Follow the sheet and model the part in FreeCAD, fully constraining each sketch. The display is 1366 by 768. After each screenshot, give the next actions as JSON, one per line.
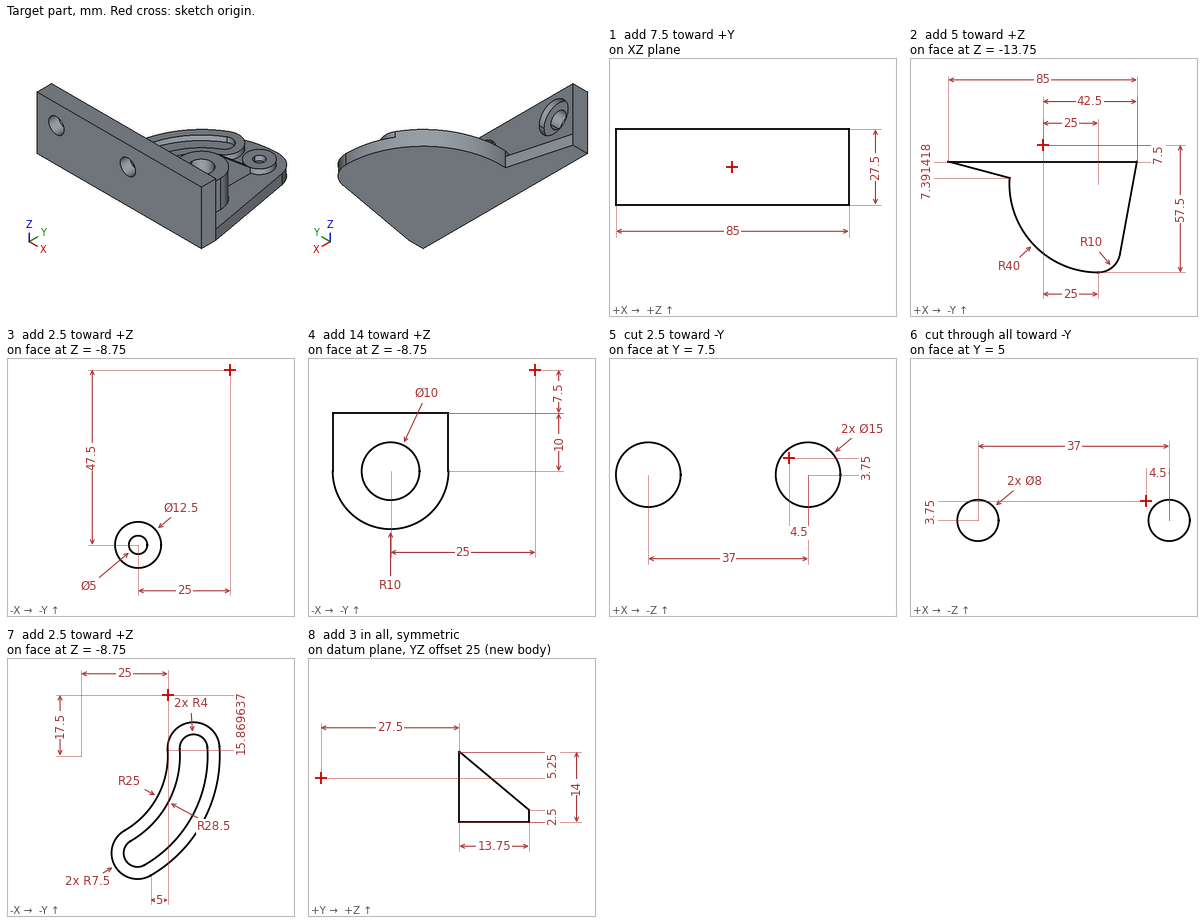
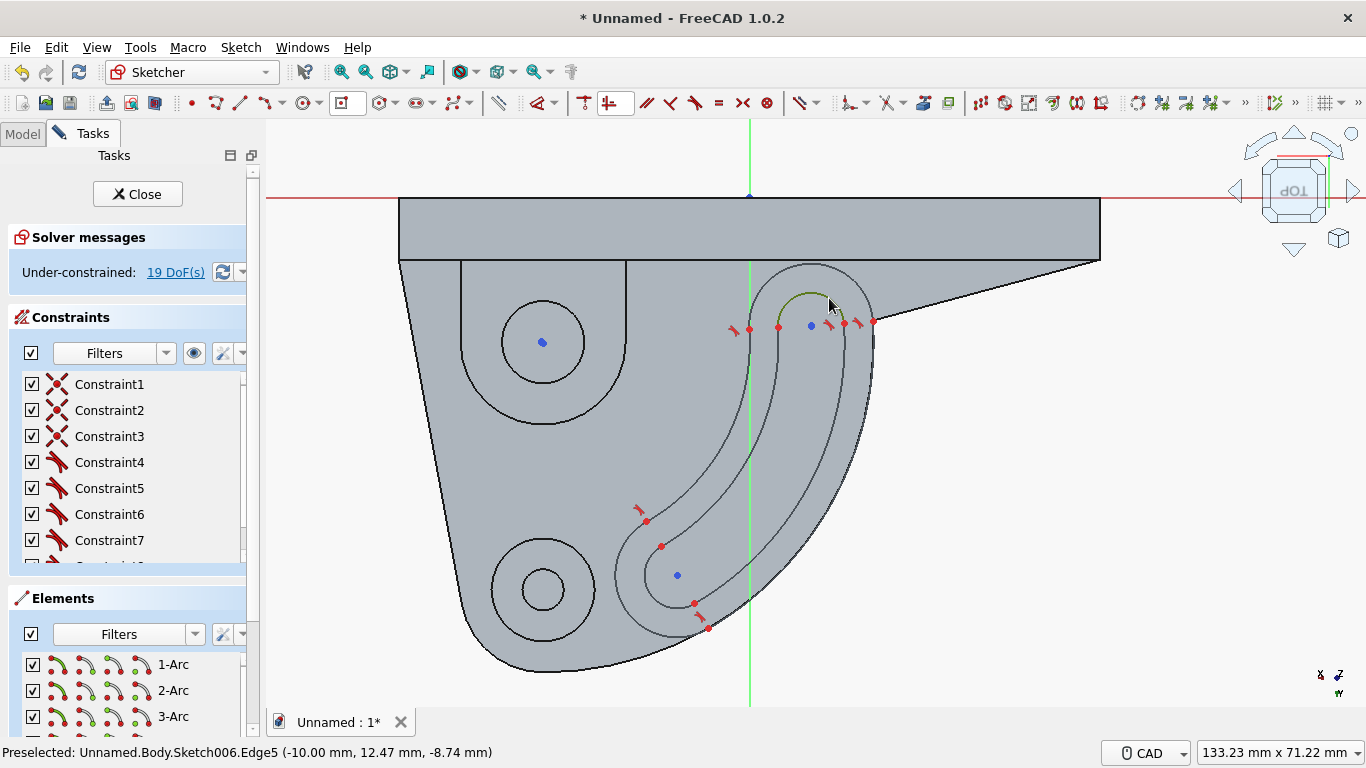
{"action": "left_click", "coordinate": [721, 497]}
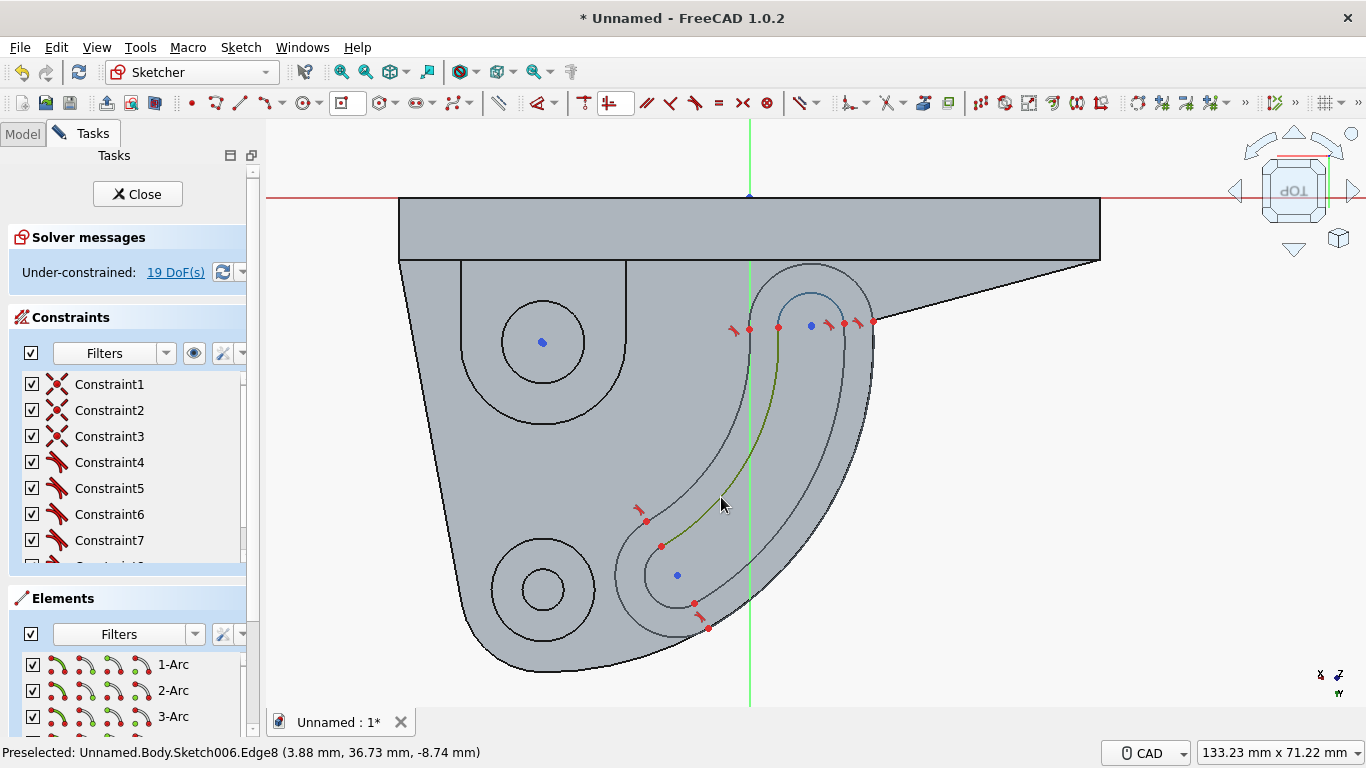
{"action": "left_click", "coordinate": [696, 104]}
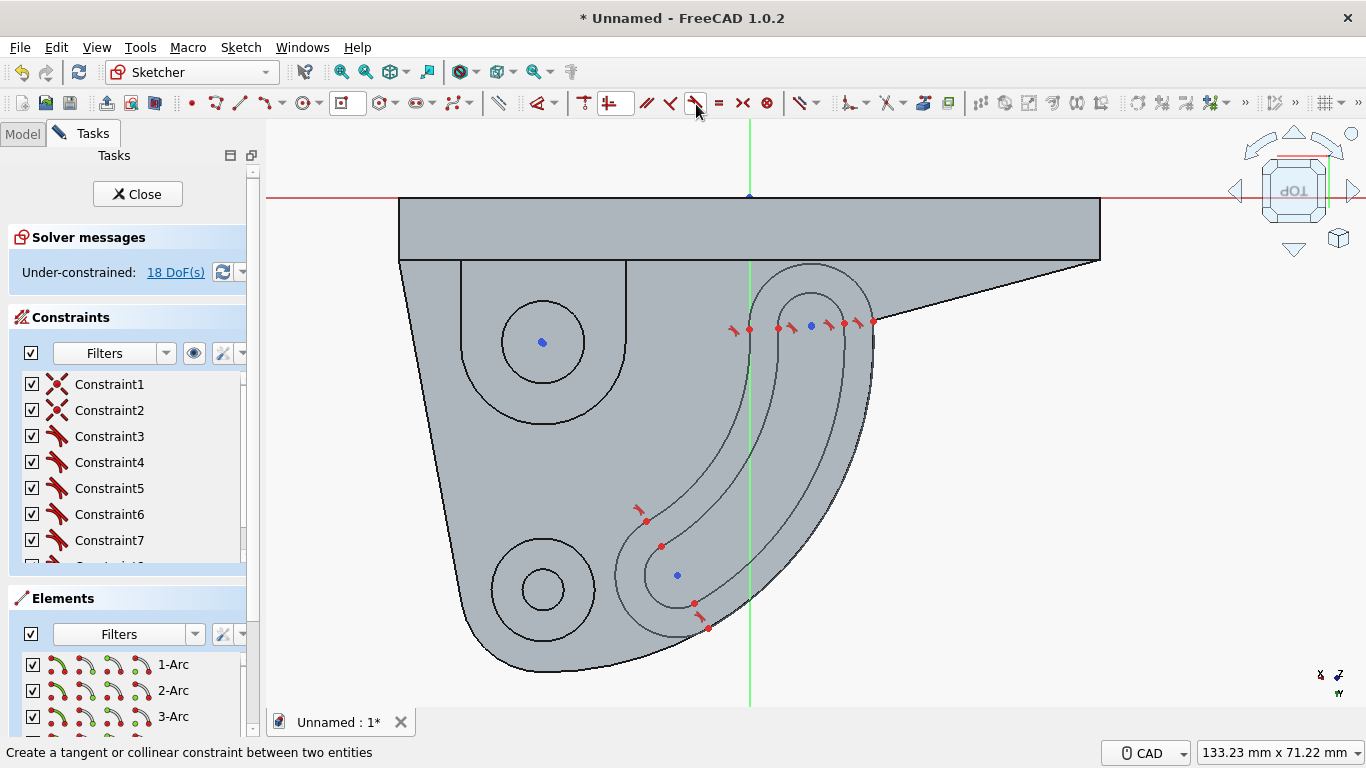
{"action": "left_click", "coordinate": [771, 540]}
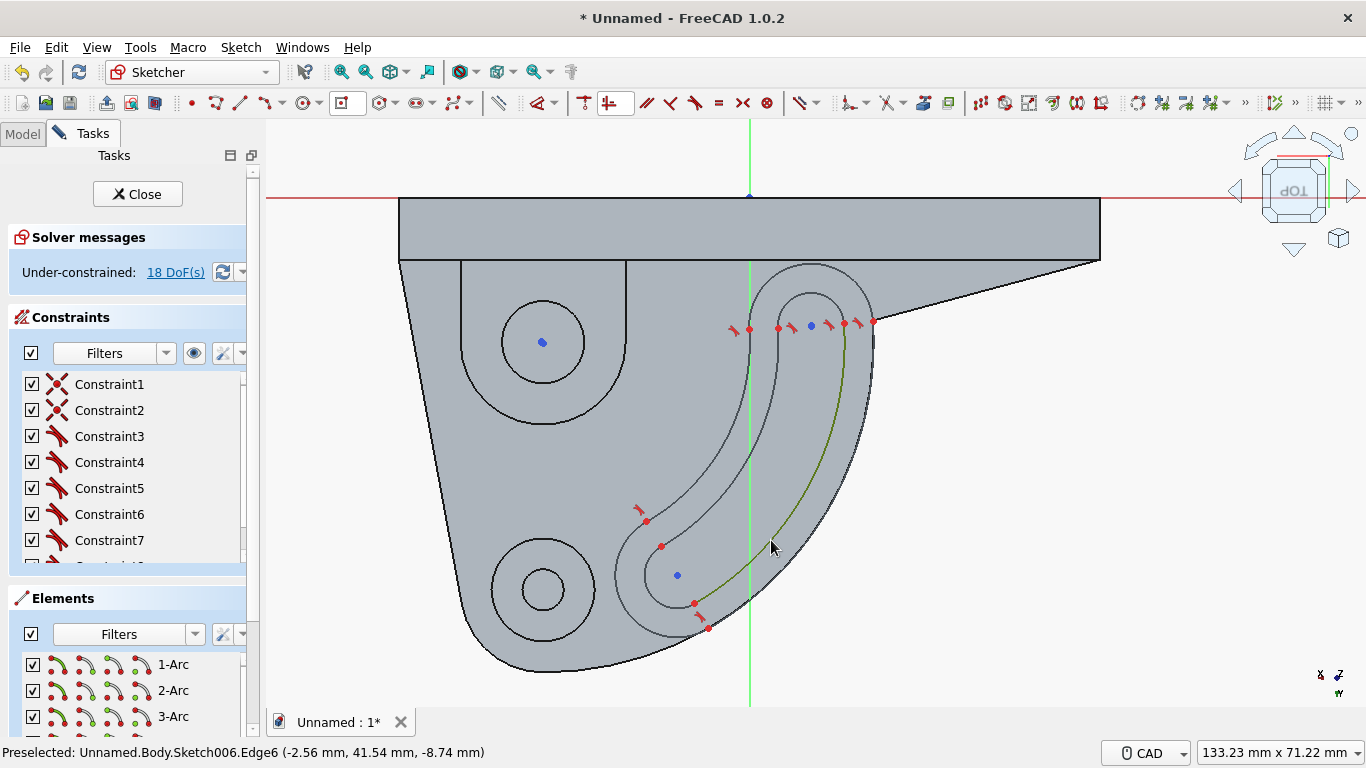
{"action": "left_click", "coordinate": [645, 572]}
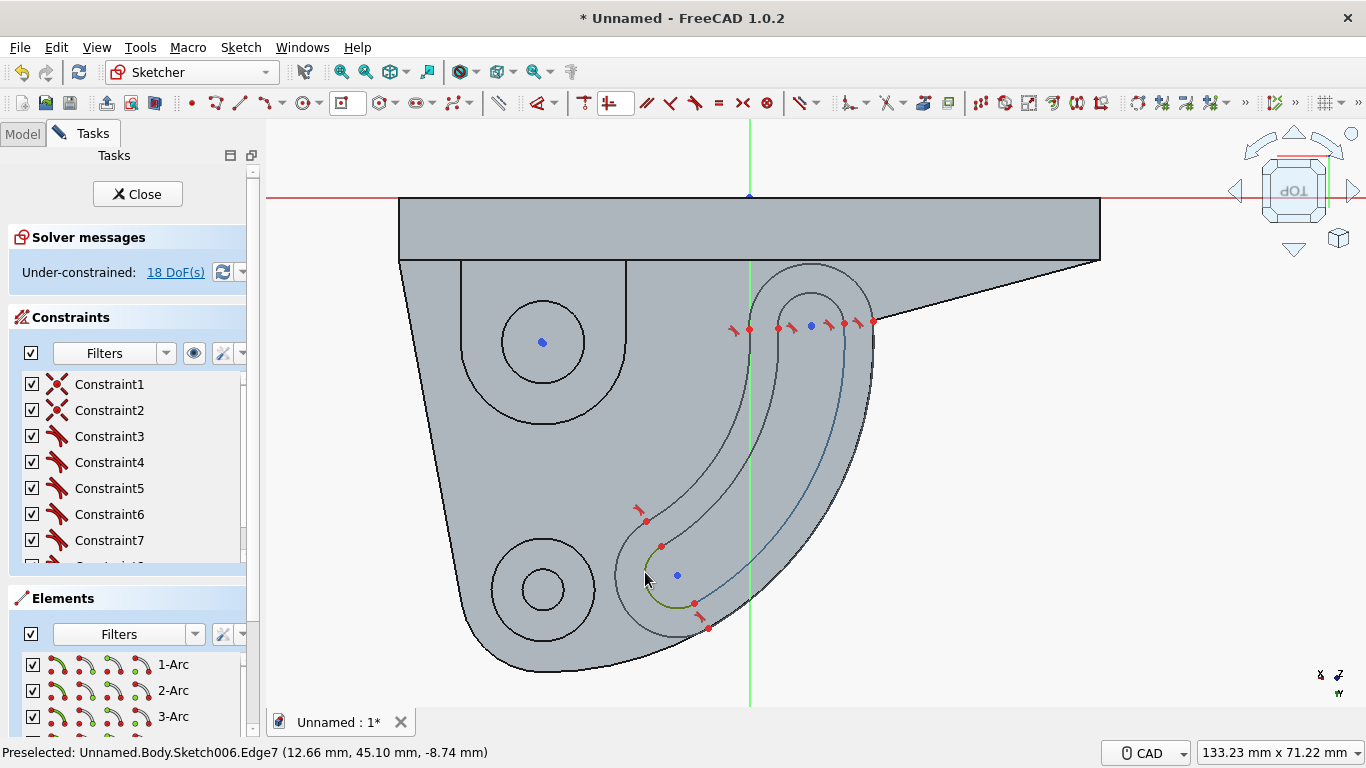
{"action": "left_click", "coordinate": [696, 104]}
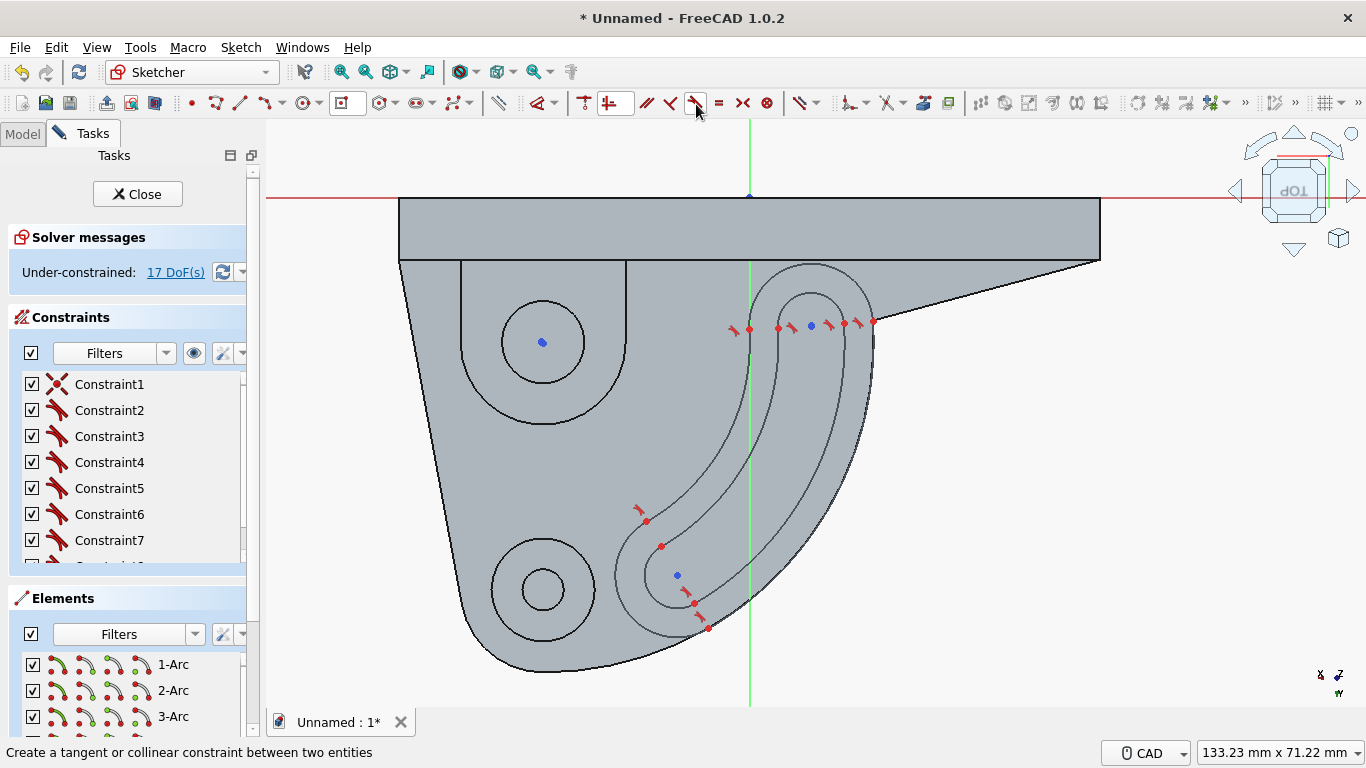
{"action": "left_click", "coordinate": [645, 572]}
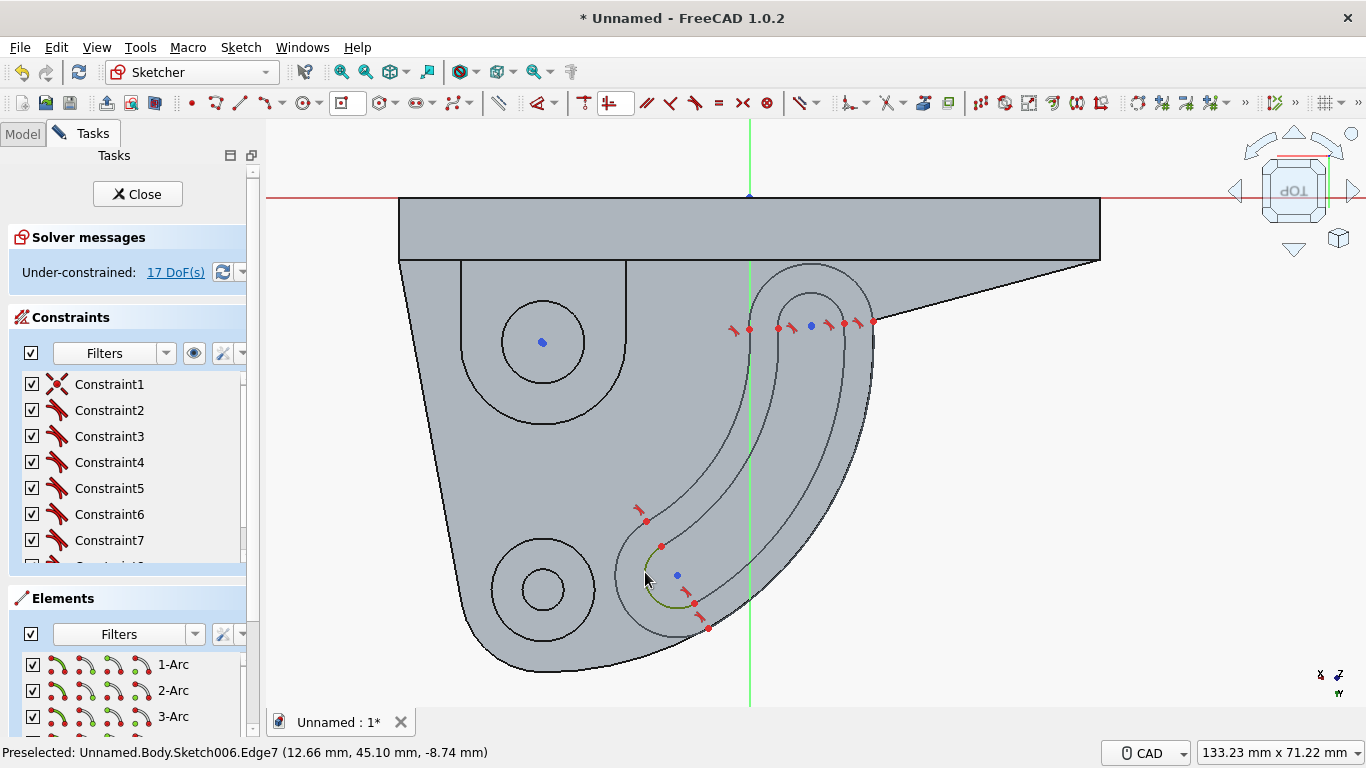
{"action": "left_click", "coordinate": [721, 497]}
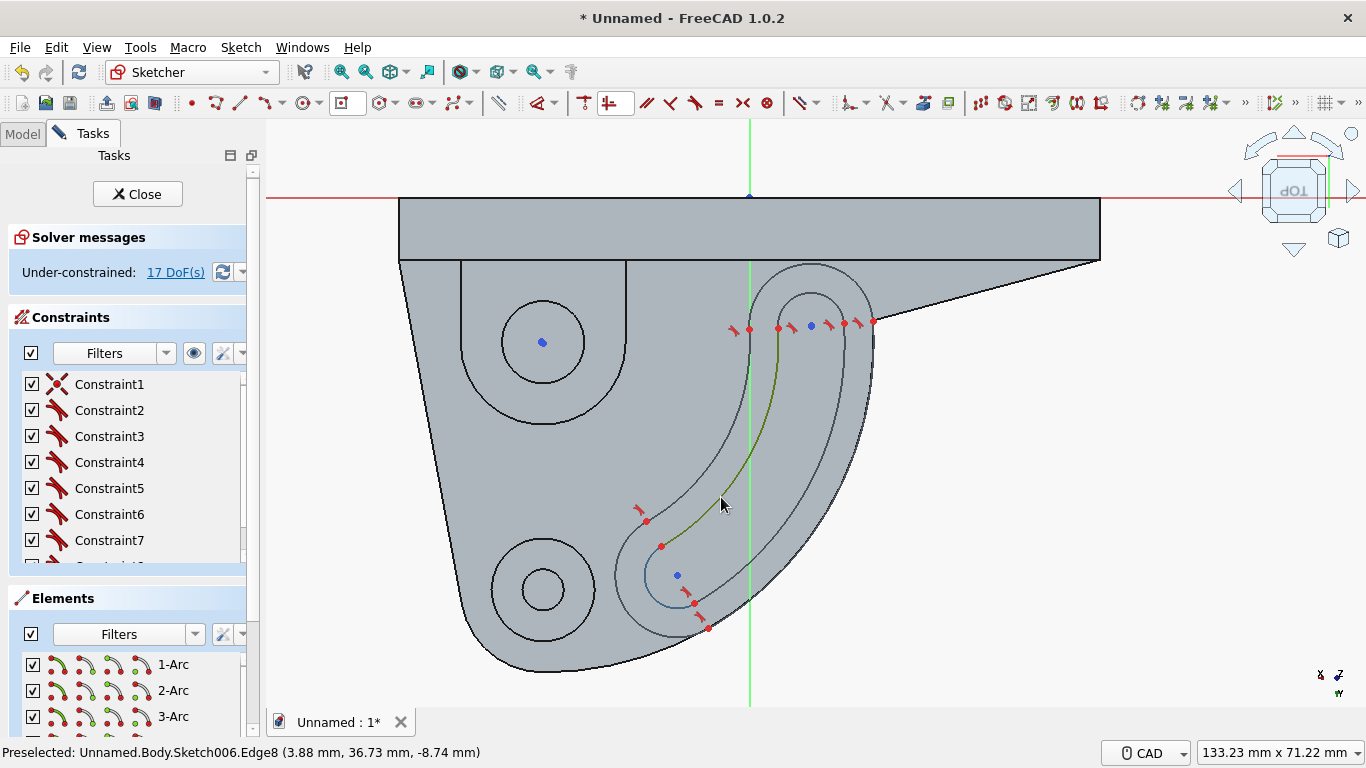
{"action": "left_click", "coordinate": [696, 104]}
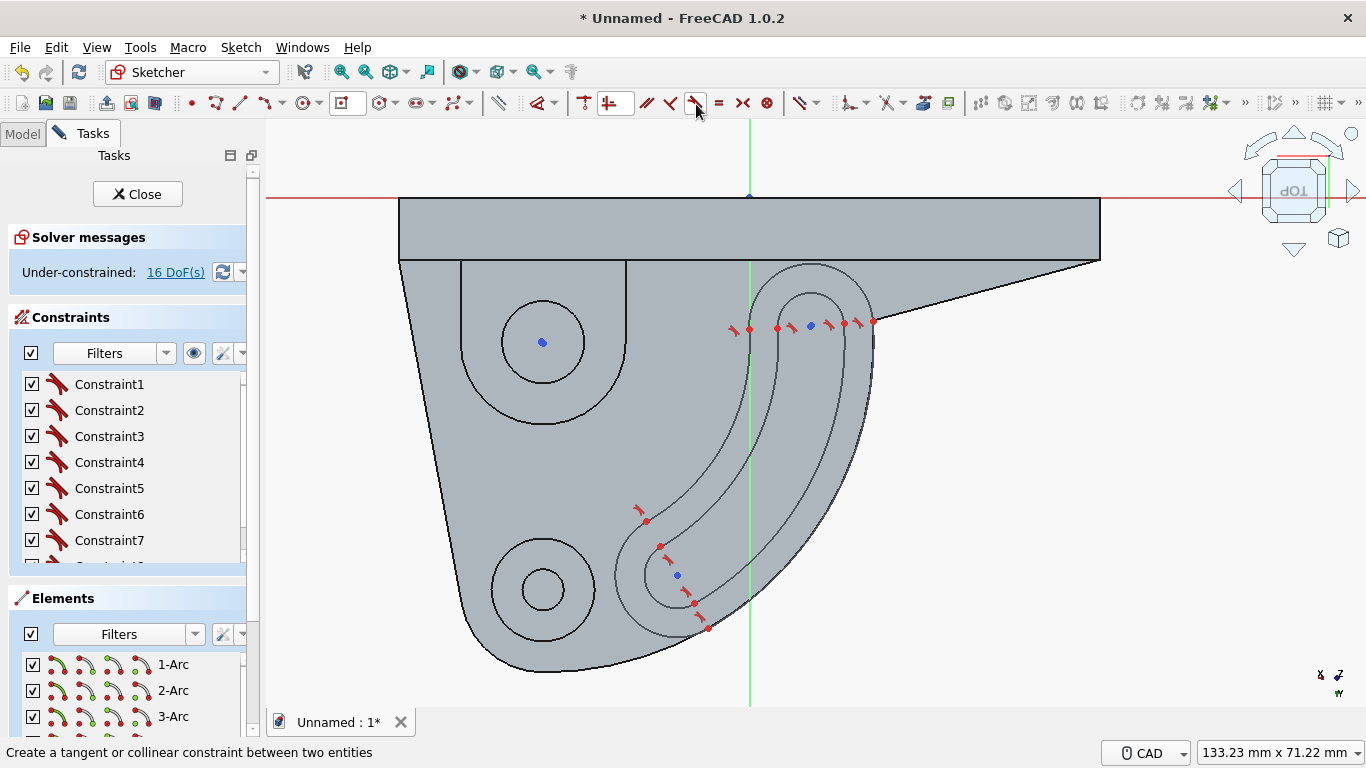
{"action": "left_click", "coordinate": [699, 478]}